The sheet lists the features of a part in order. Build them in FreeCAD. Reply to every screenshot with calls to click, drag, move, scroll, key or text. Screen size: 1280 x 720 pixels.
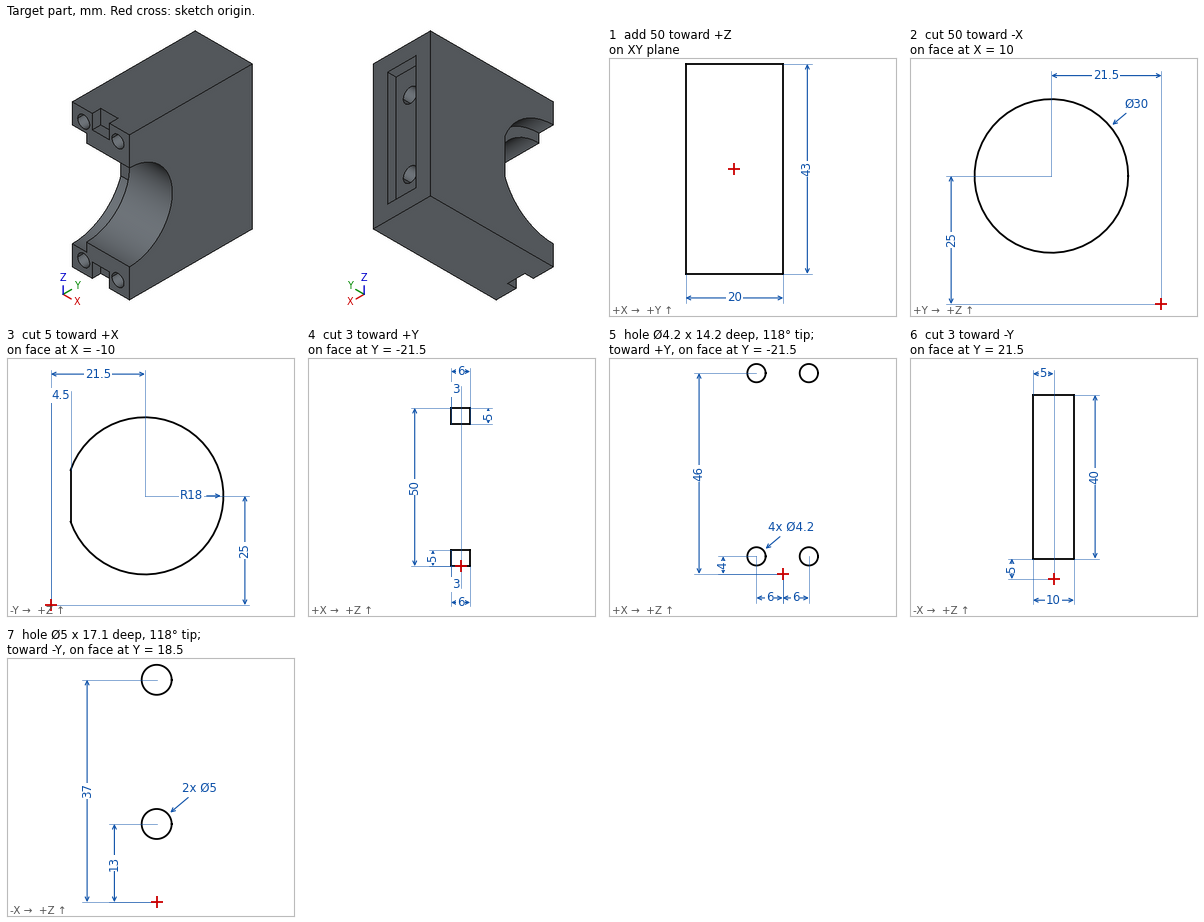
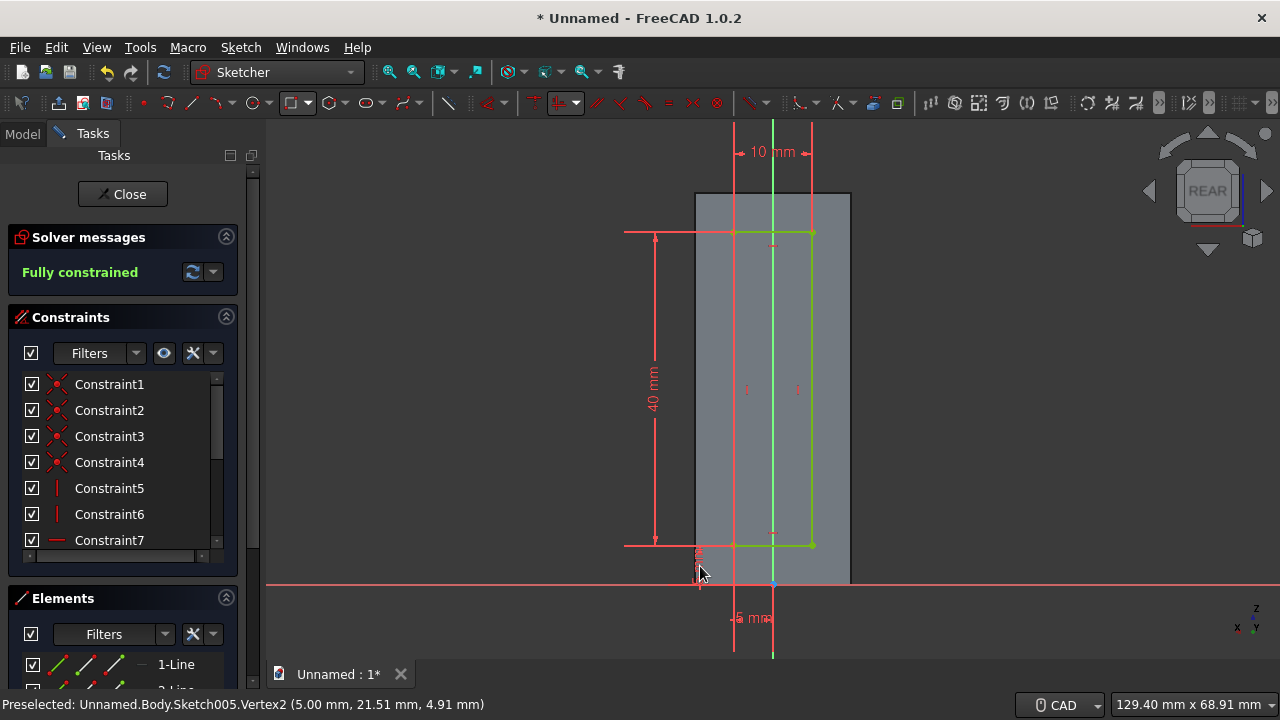
click(123, 194)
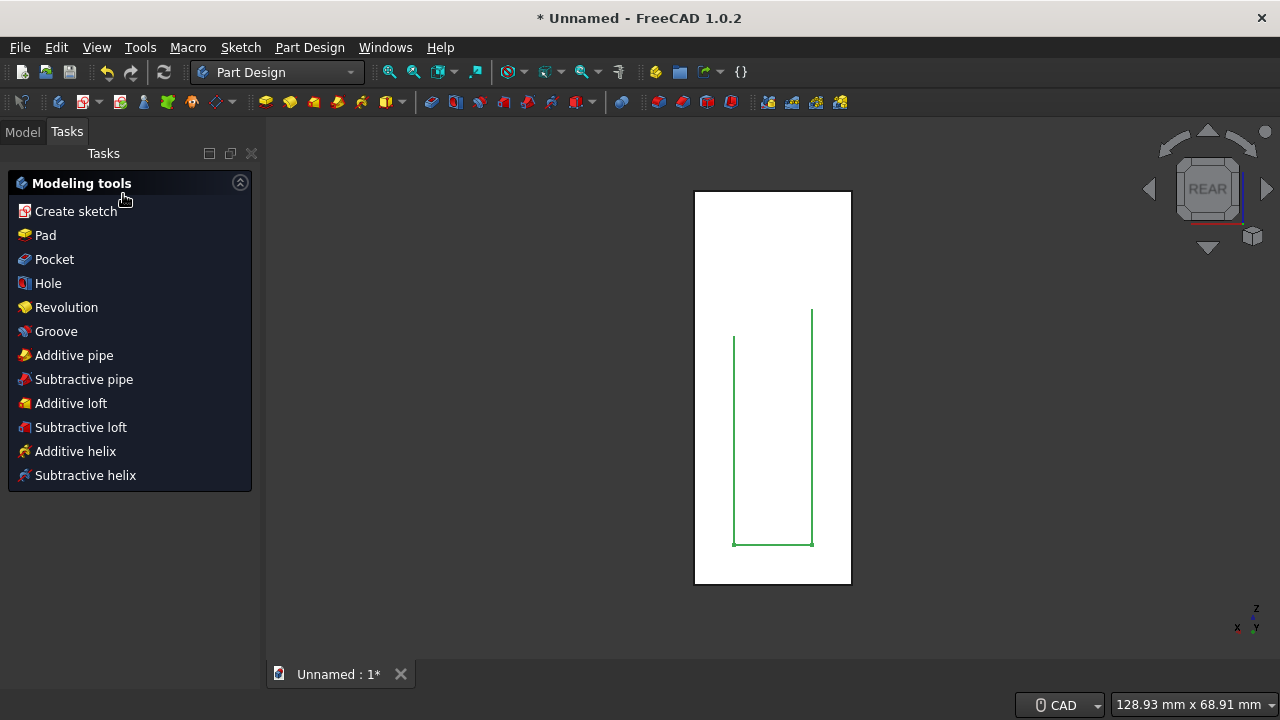
click(432, 102)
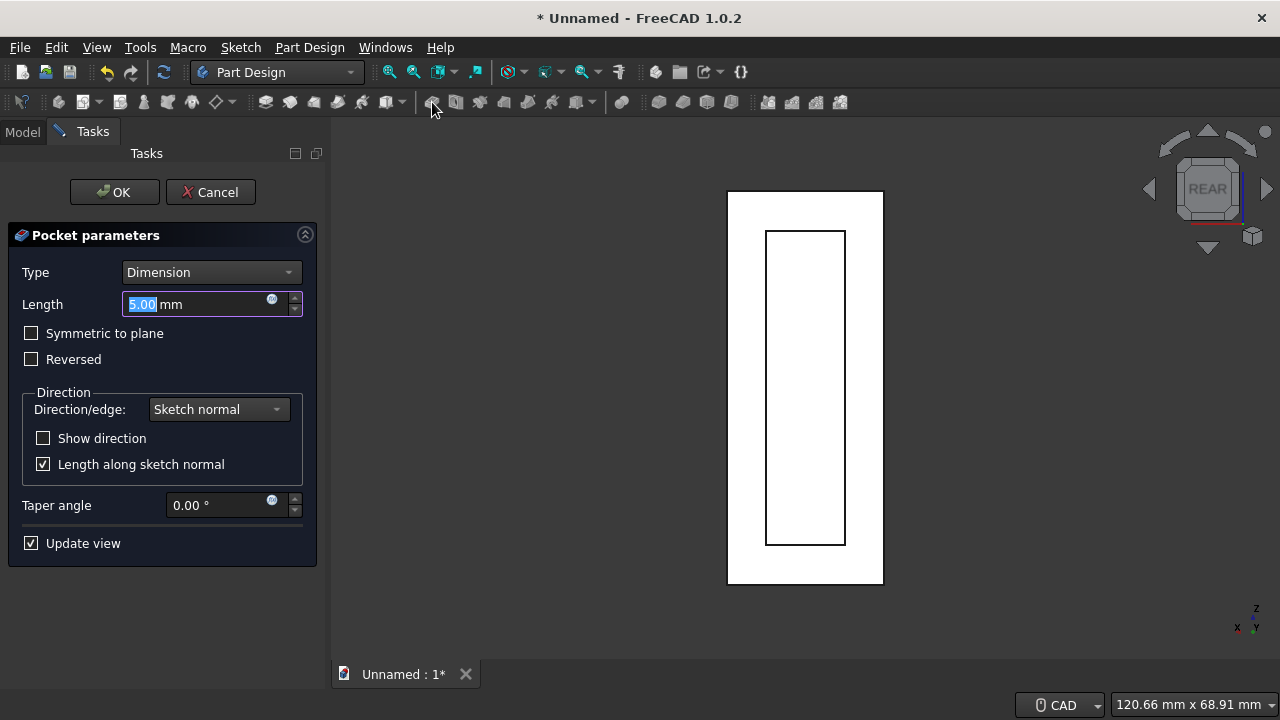
text(3)
key(Tab)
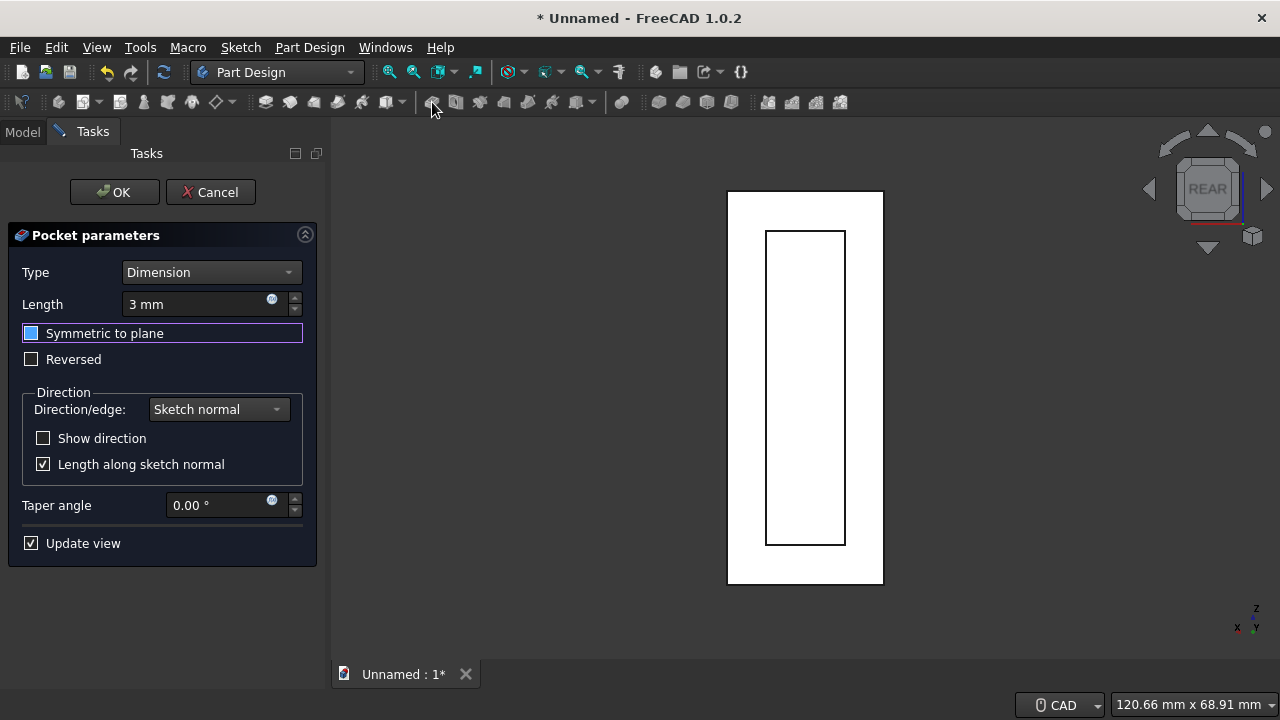
click(115, 192)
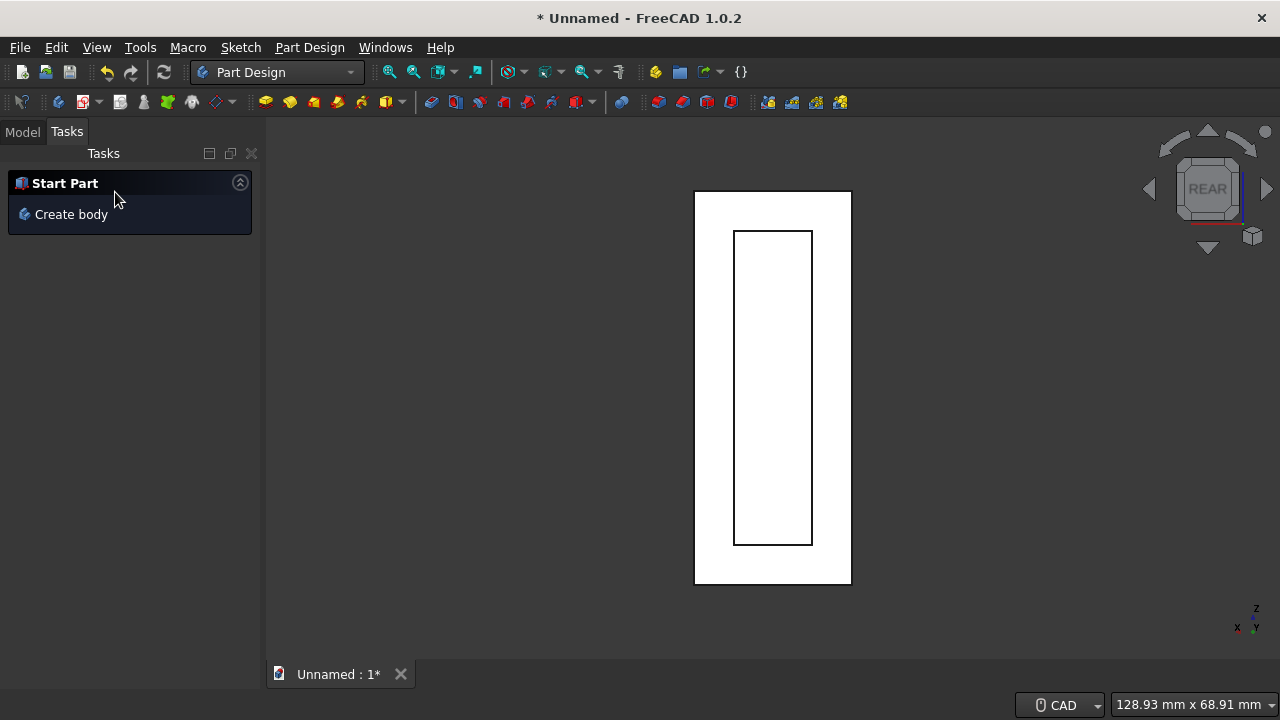
click(773, 297)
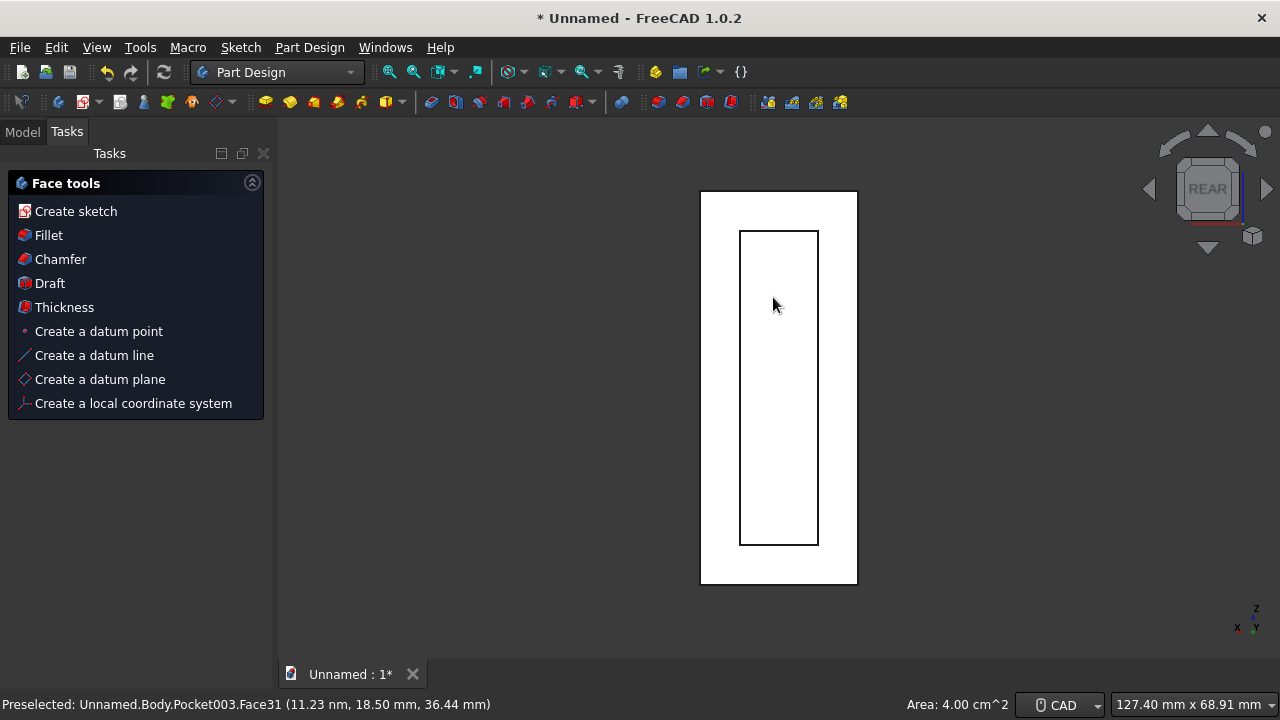
click(84, 102)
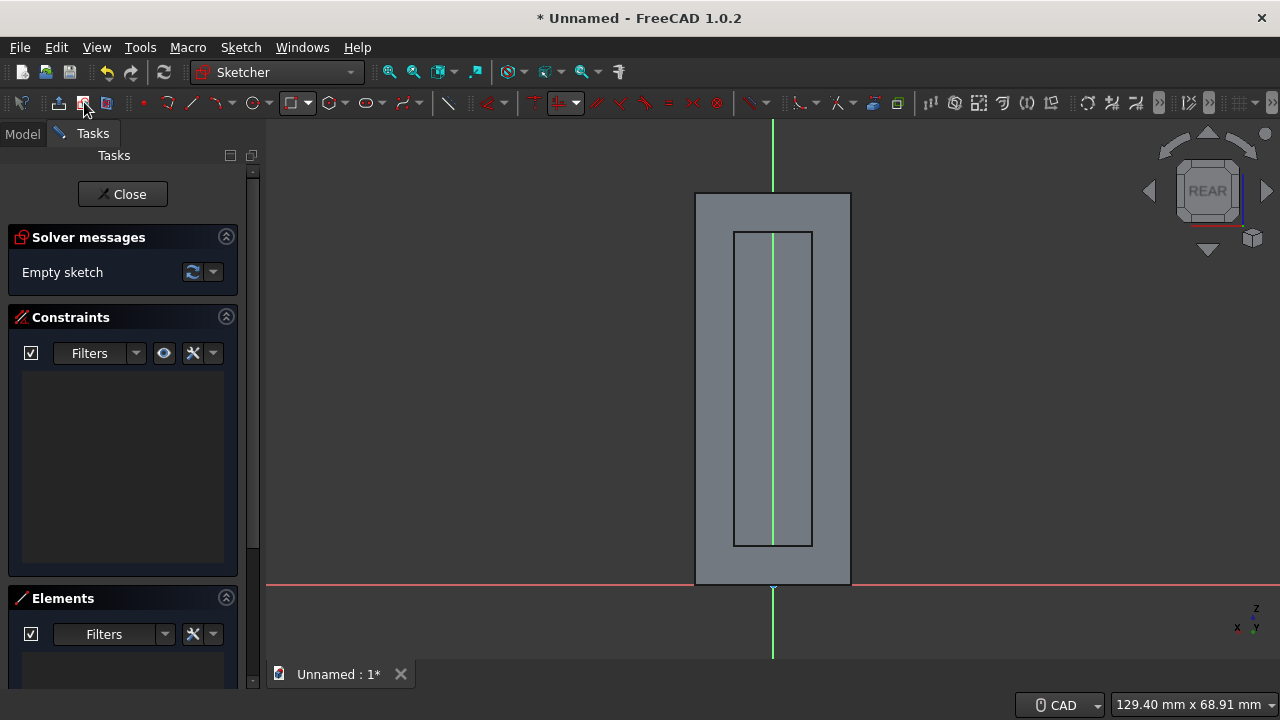
click(254, 104)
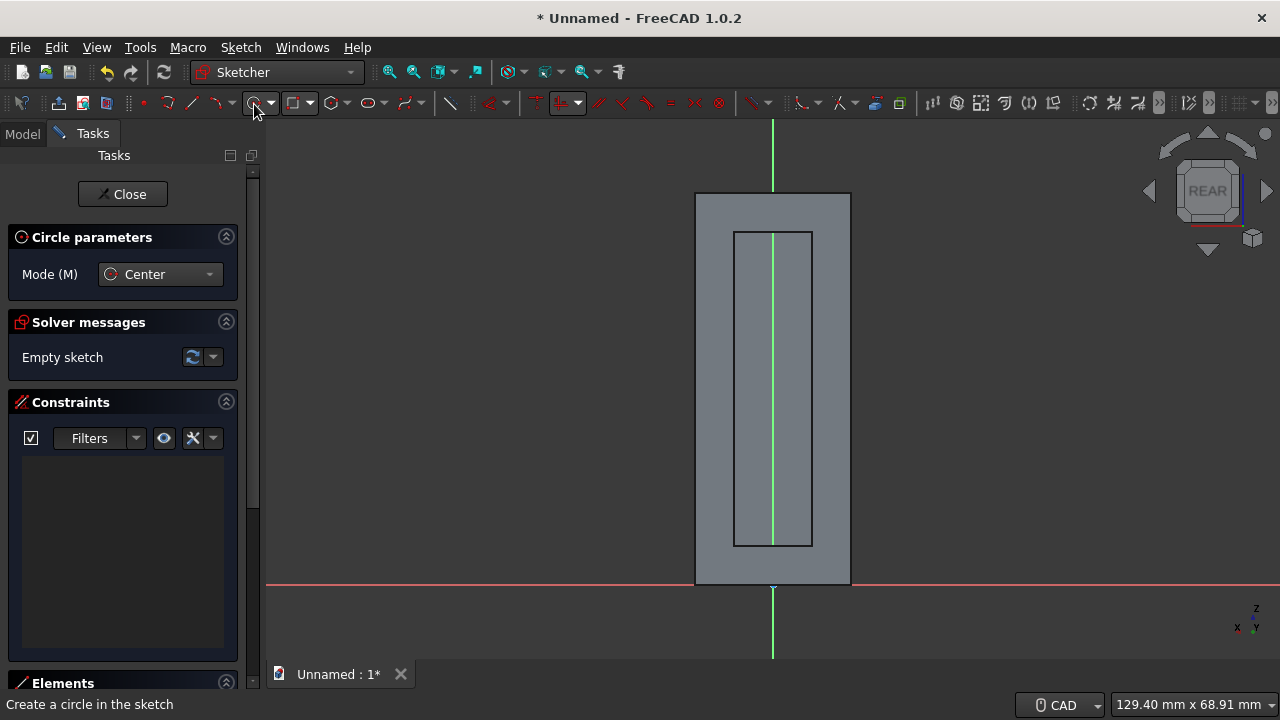
click(773, 483)
move(791, 476)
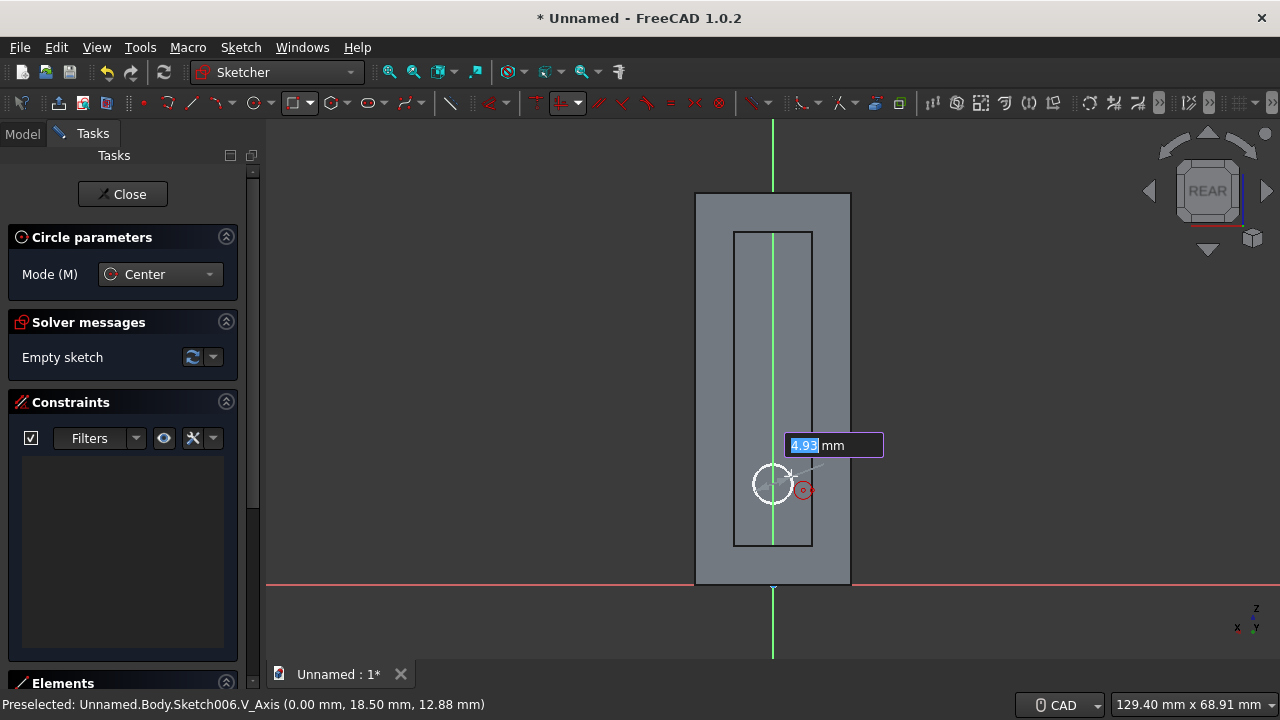
text(5)
key(Return)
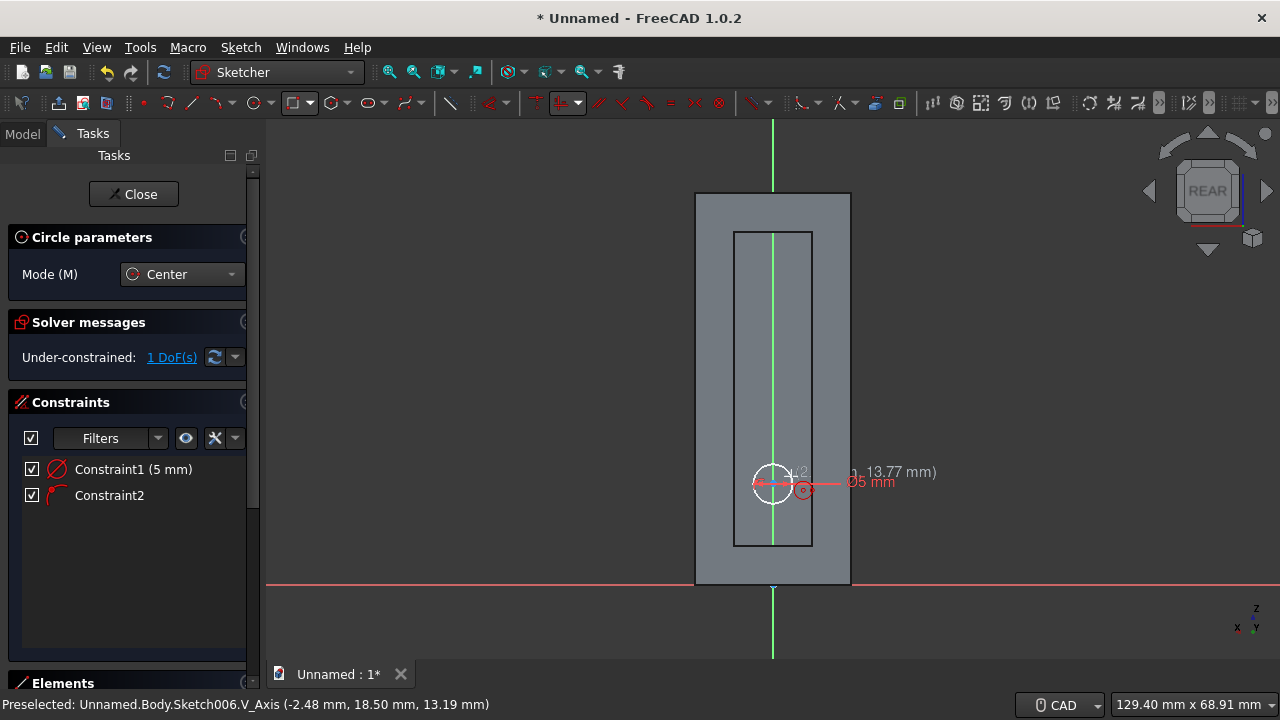
click(773, 295)
move(791, 288)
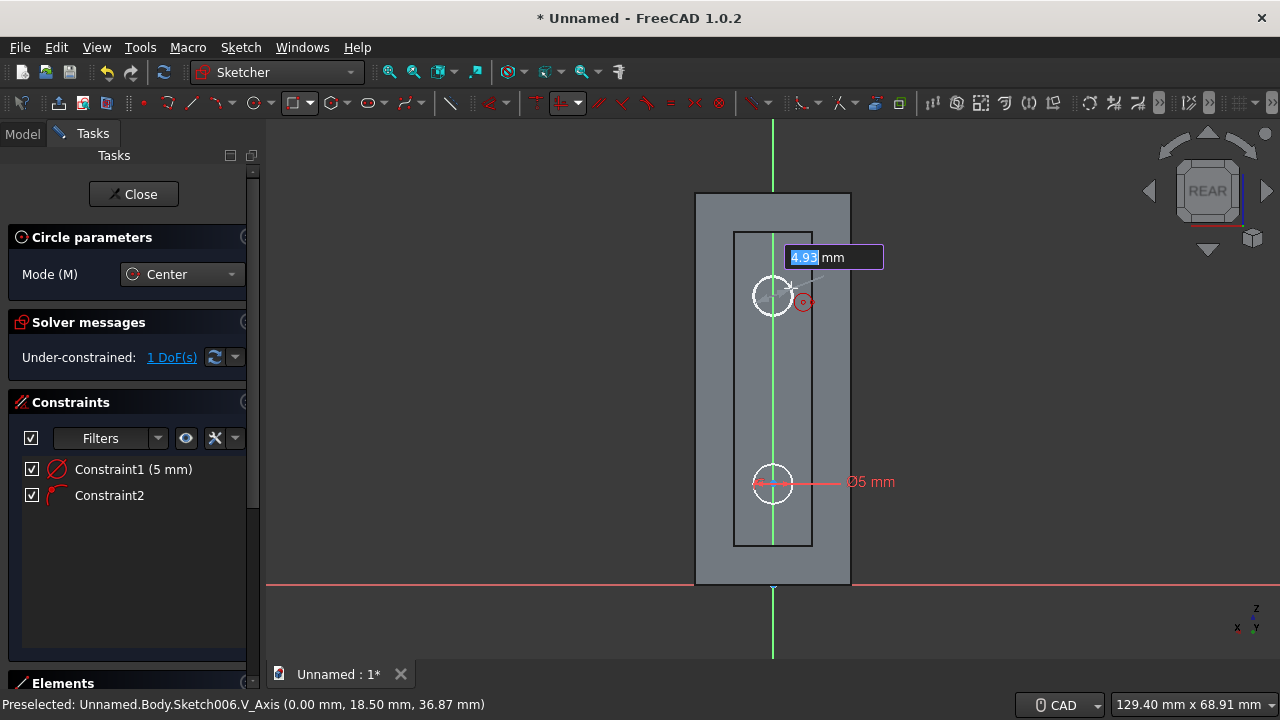
text(5)
key(Return)
key(Escape)